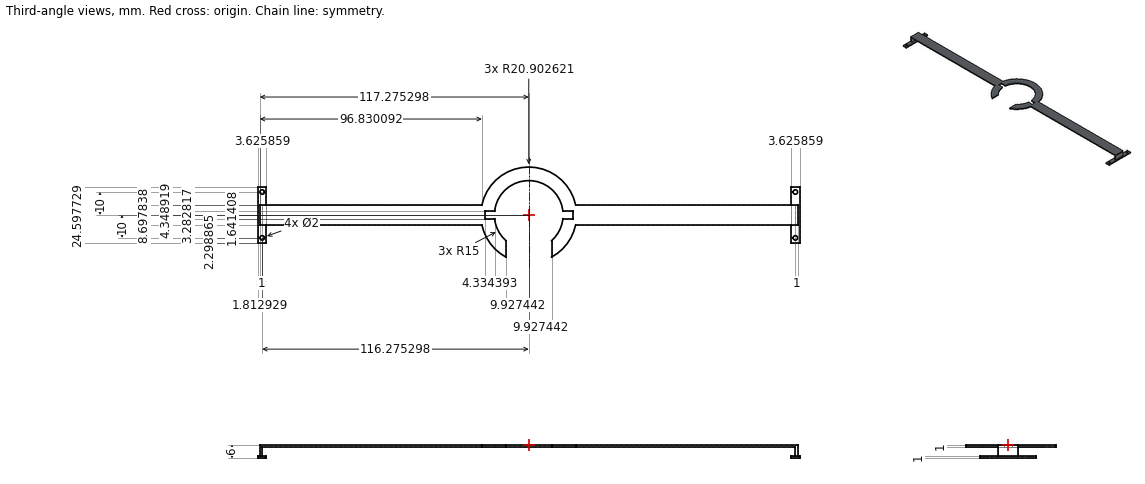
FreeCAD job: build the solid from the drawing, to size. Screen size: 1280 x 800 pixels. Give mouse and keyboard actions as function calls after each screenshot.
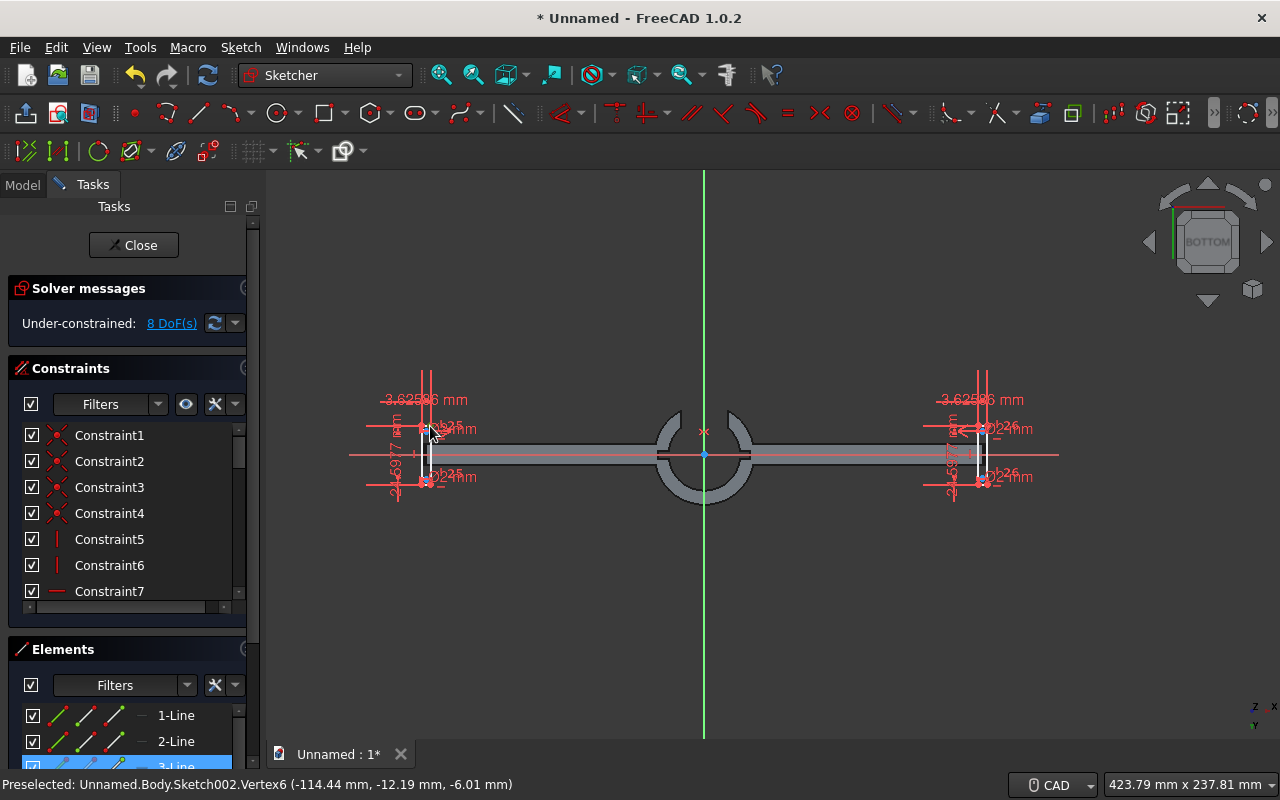
scroll(978, 426, up, 3)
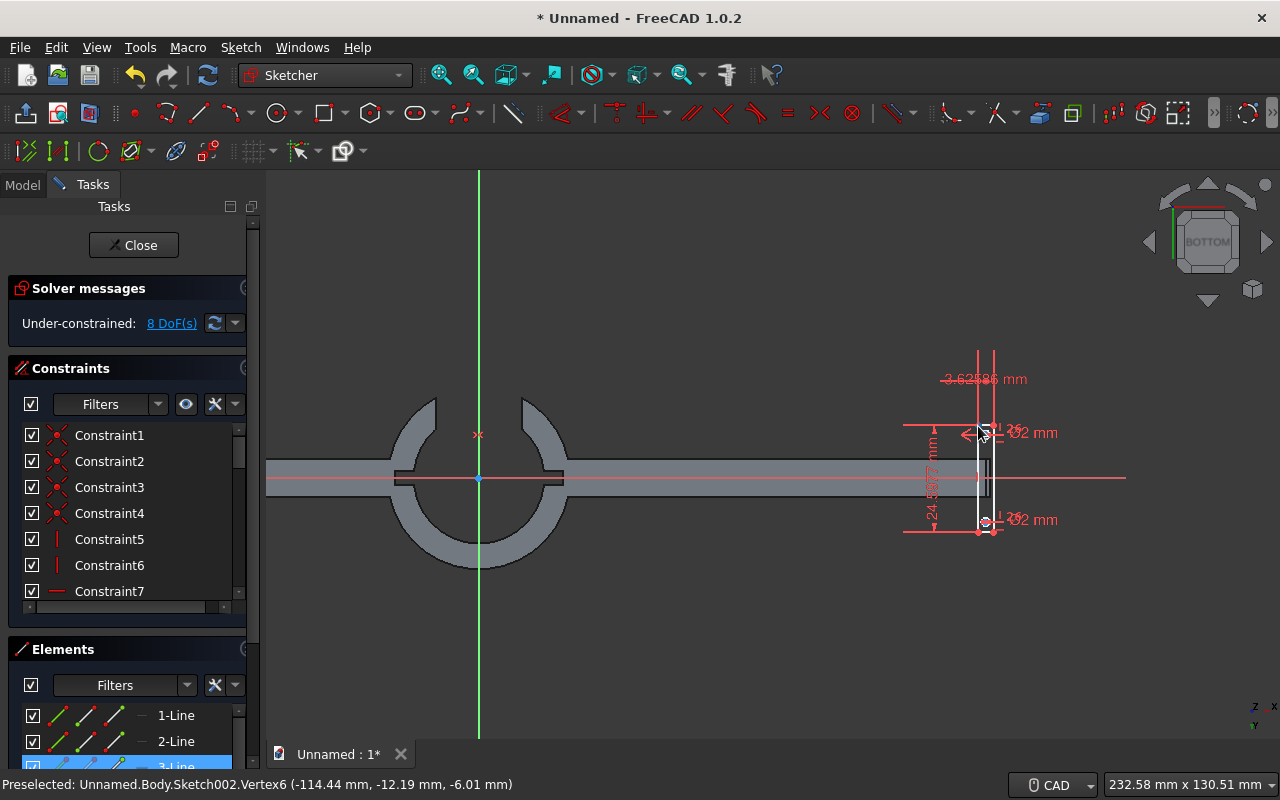
click(978, 425)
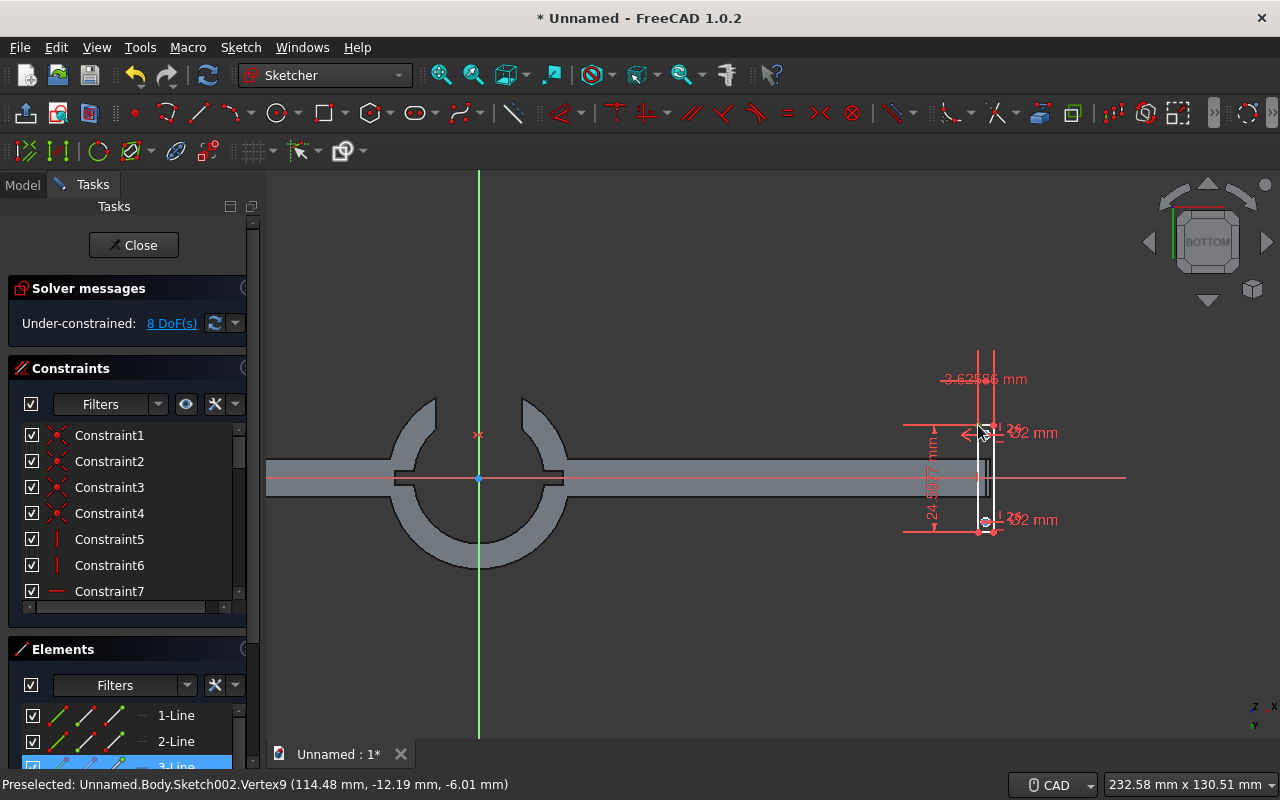
click(479, 674)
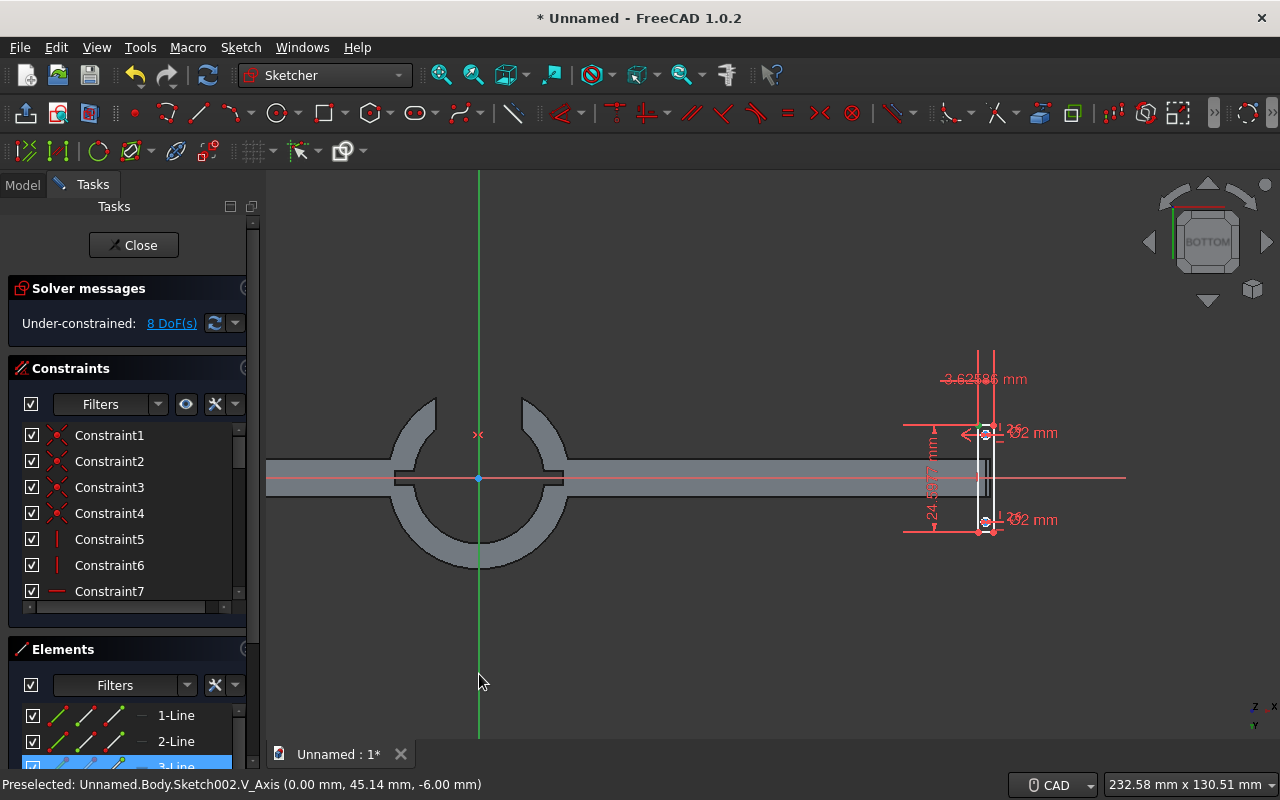
click(820, 114)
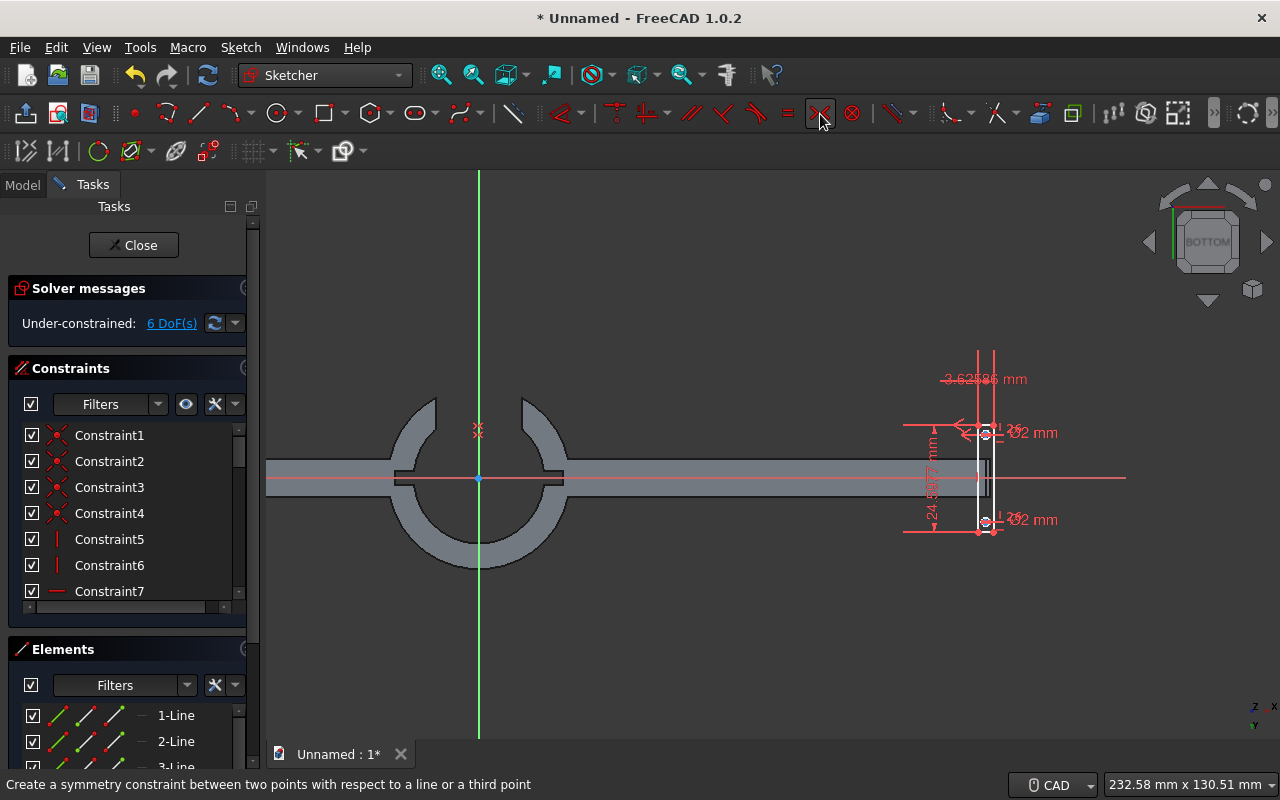
click(560, 114)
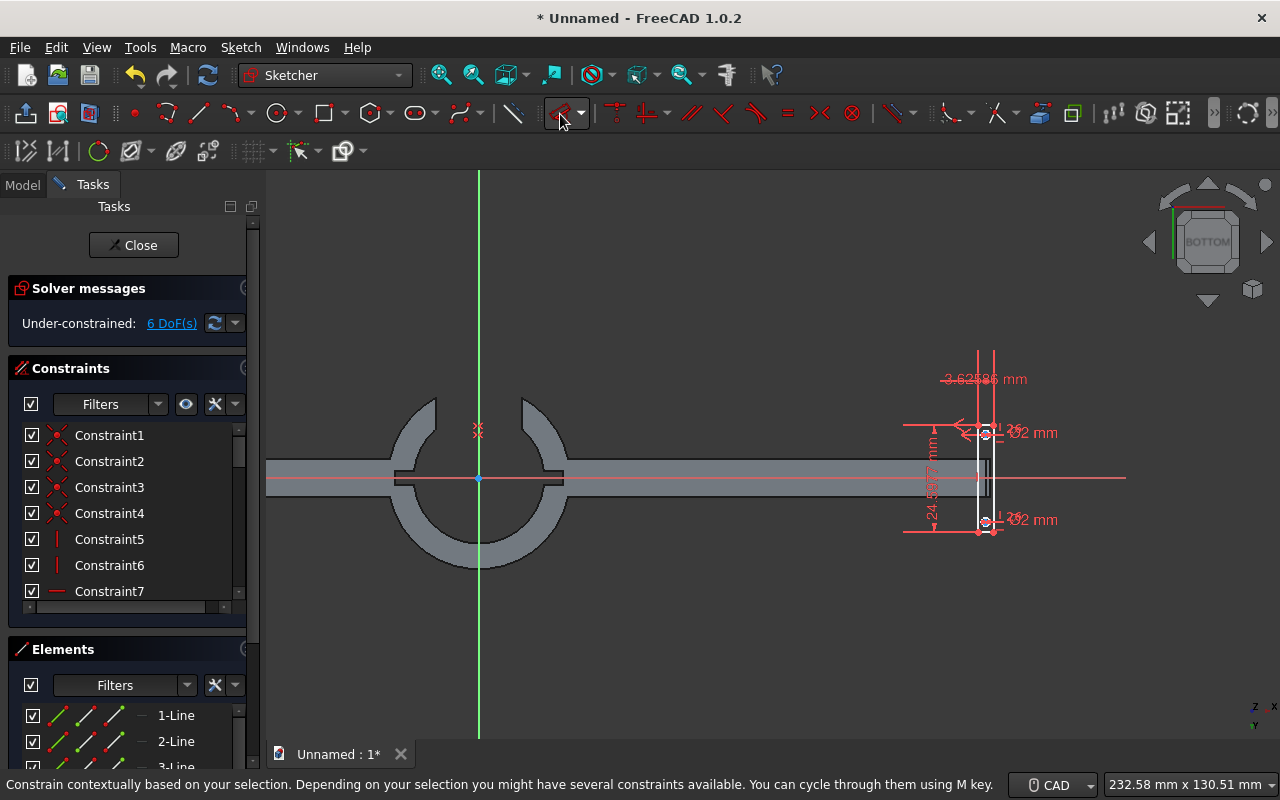
scroll(979, 426, down, 3)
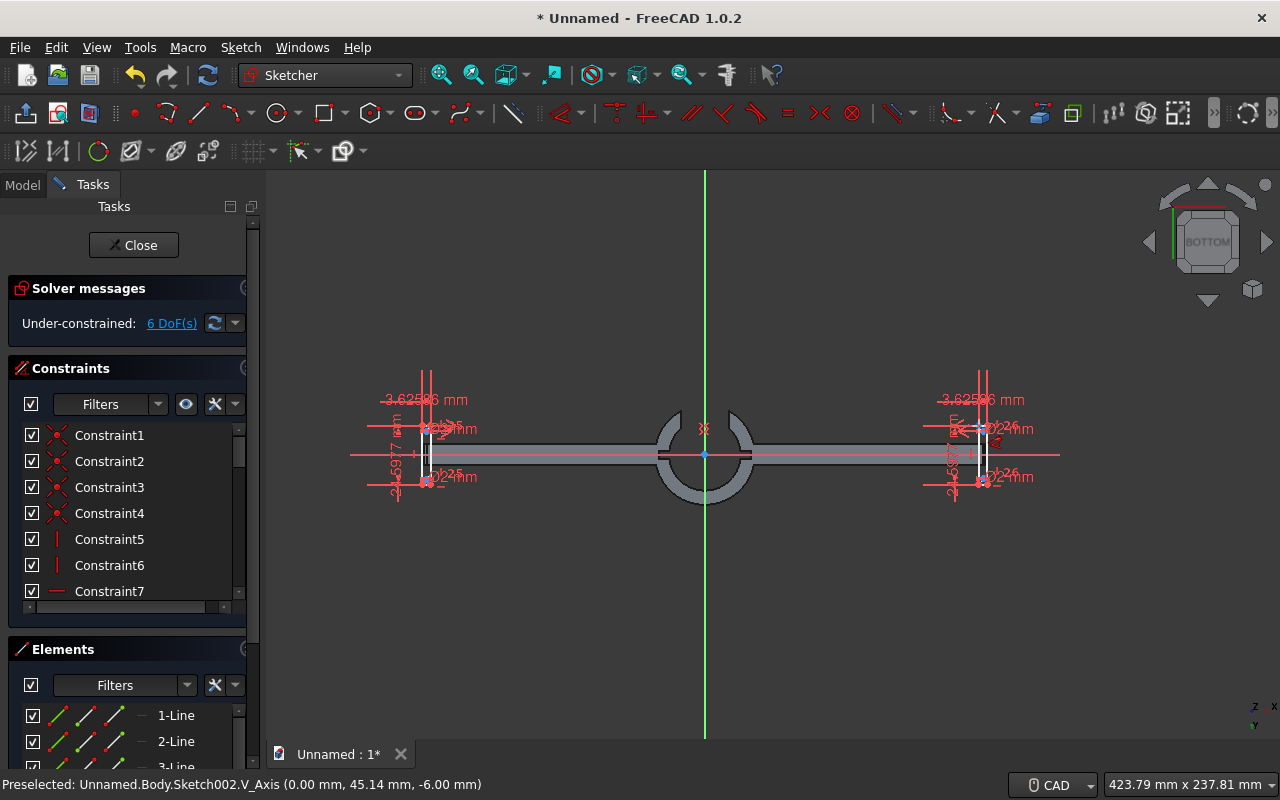
scroll(427, 431, up, 3)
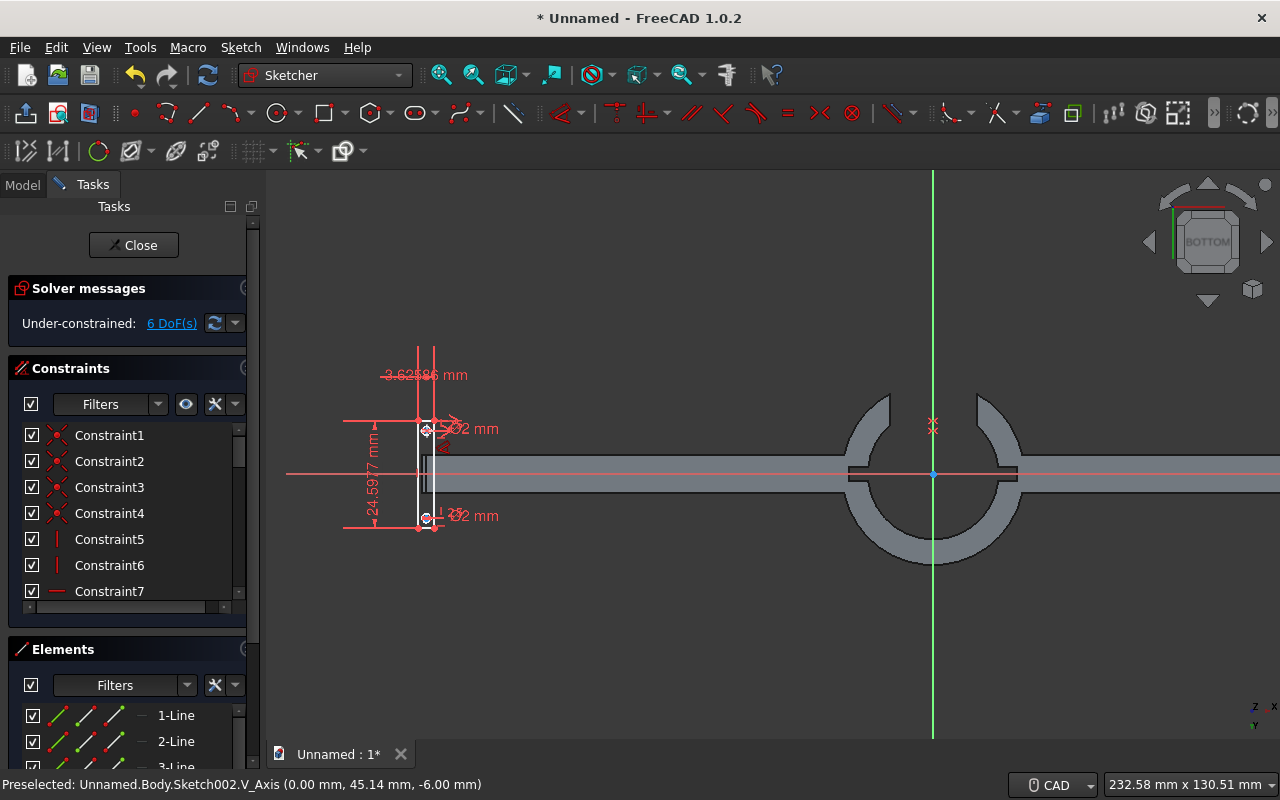
click(426, 431)
click(392, 452)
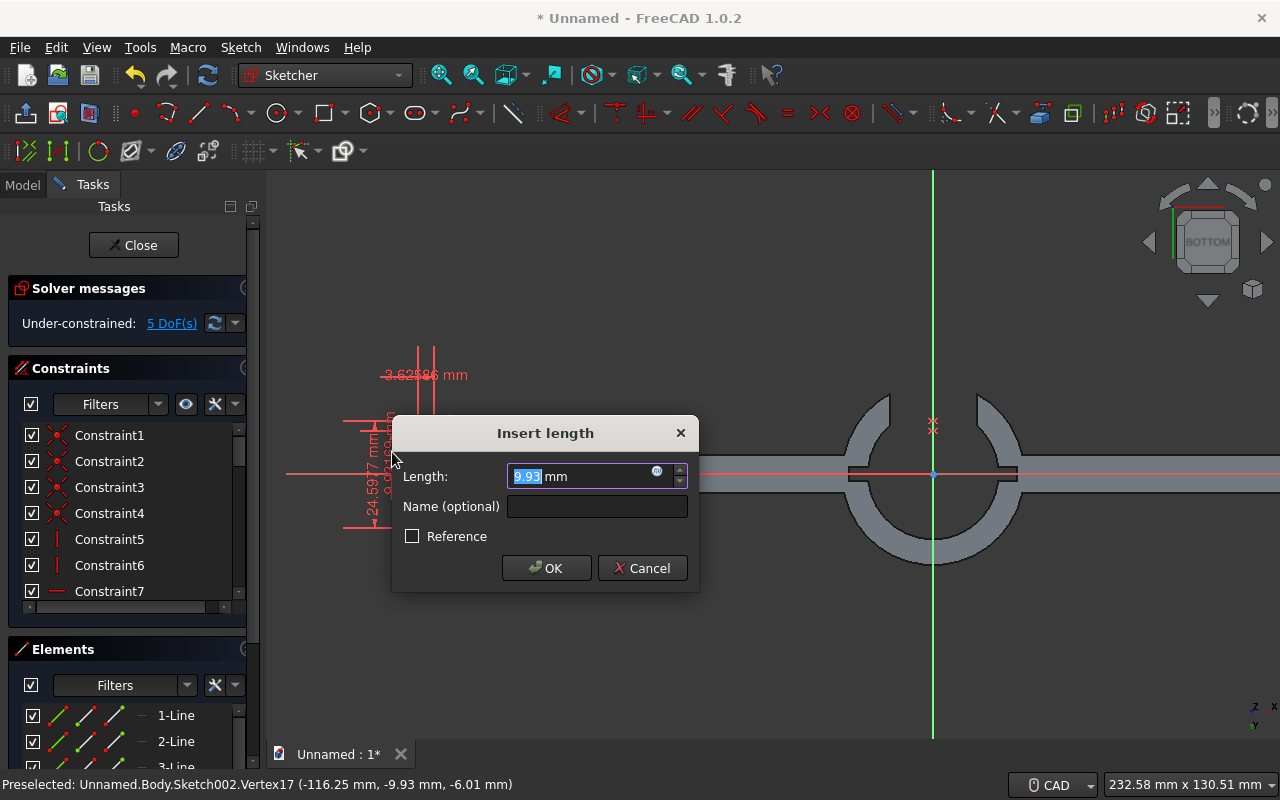
text(10)
key(Return)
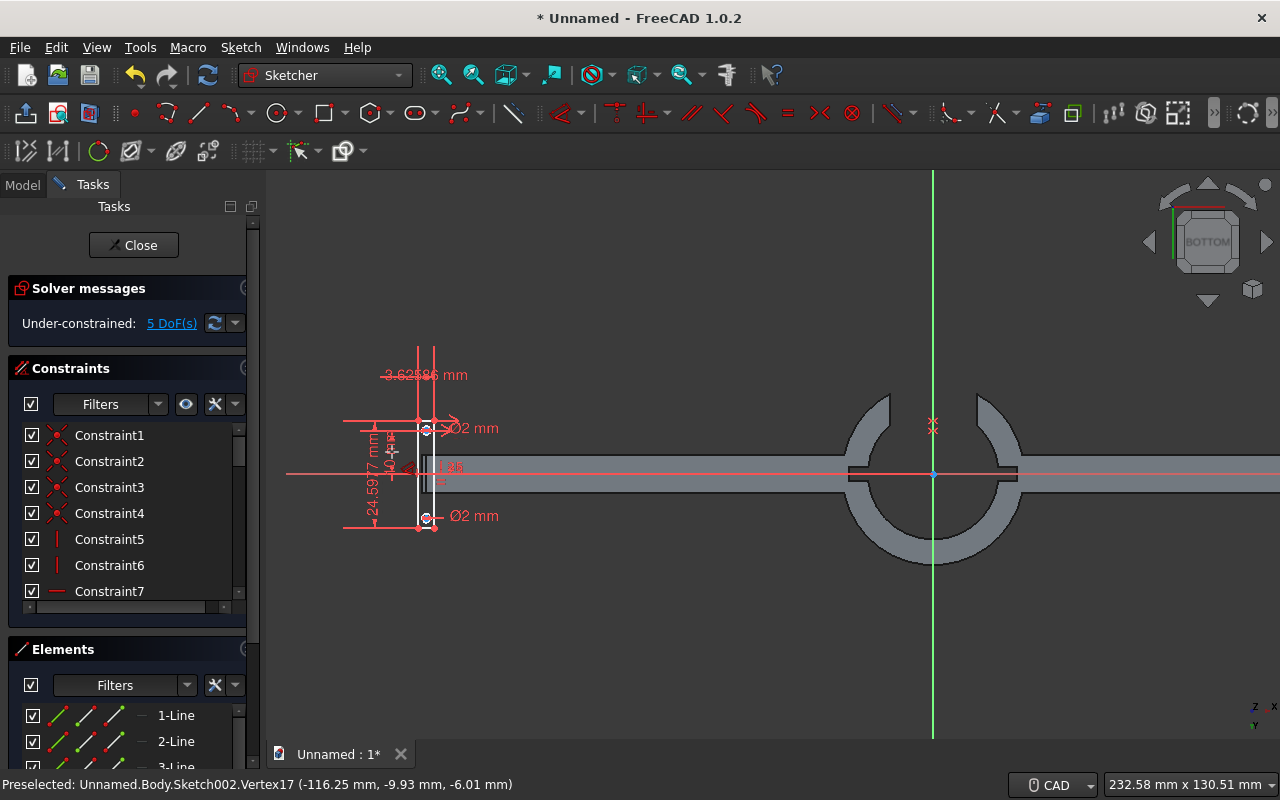
click(426, 518)
click(392, 496)